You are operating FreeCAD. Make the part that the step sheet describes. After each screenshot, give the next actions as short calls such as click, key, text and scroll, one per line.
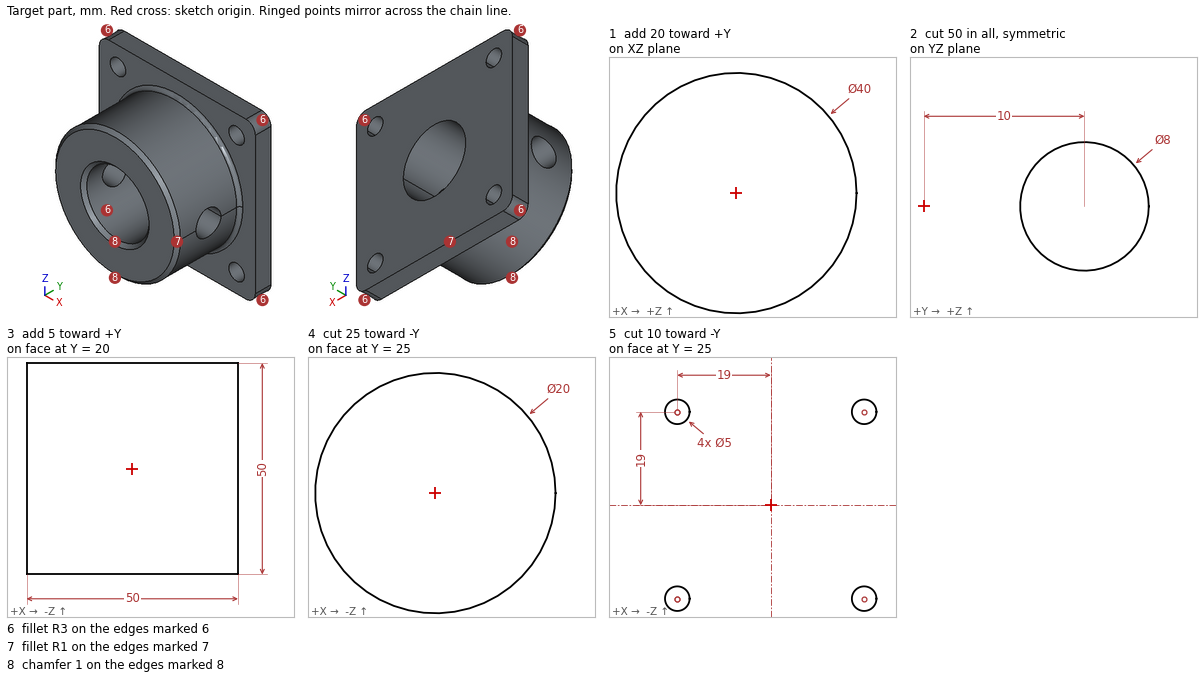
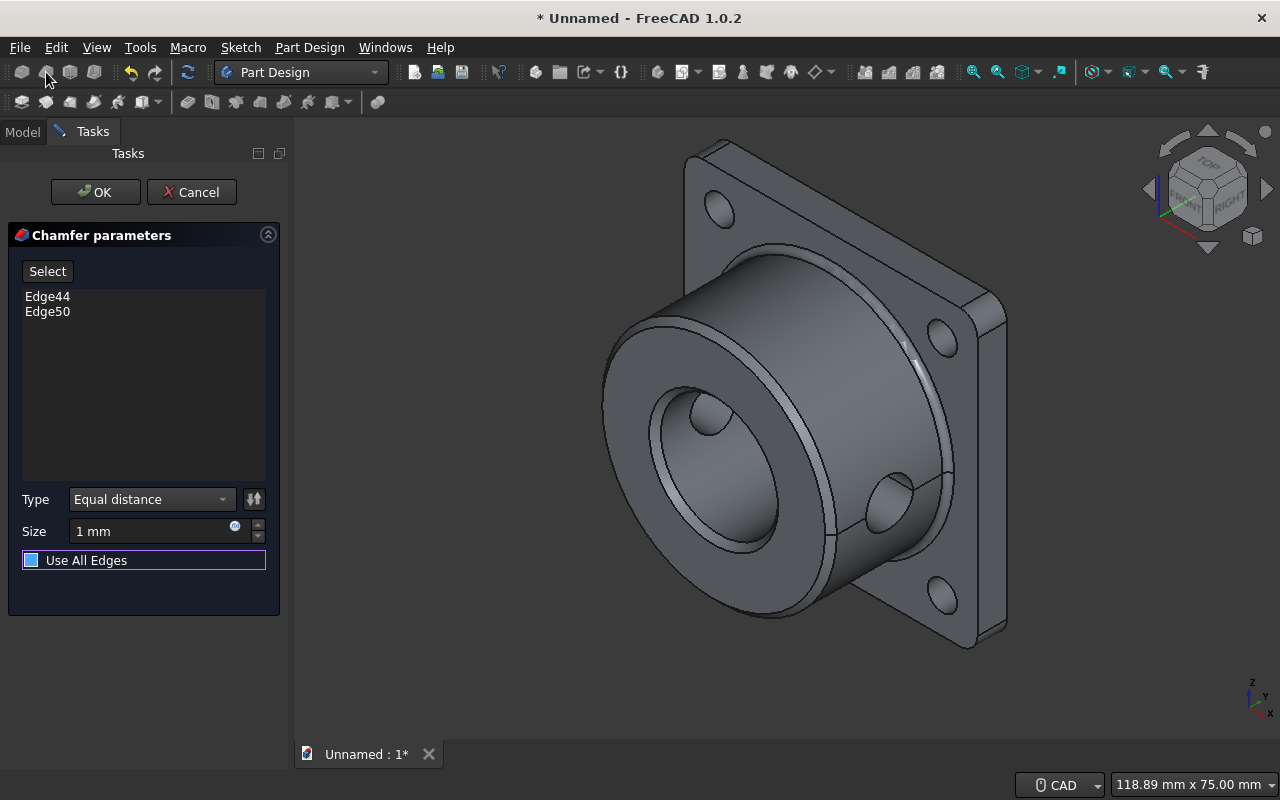
click(96, 192)